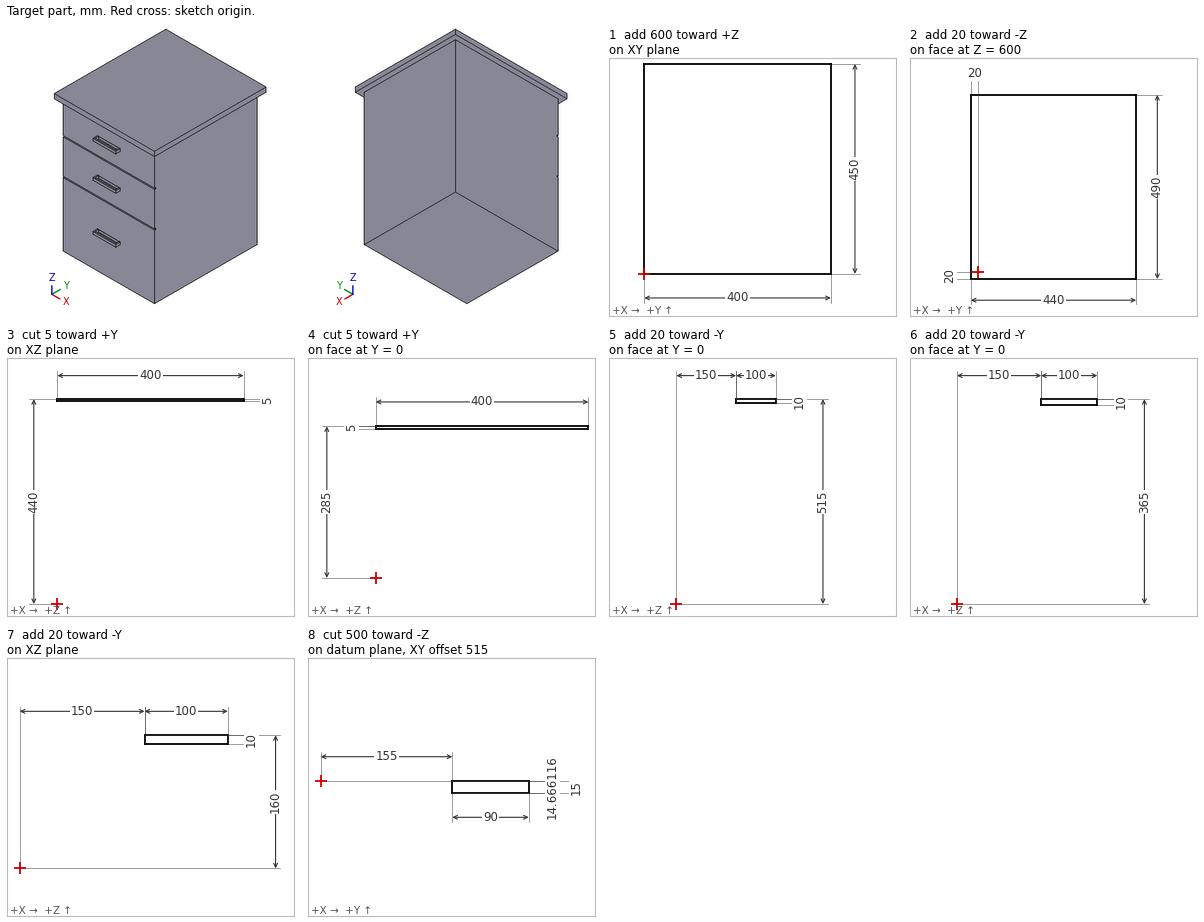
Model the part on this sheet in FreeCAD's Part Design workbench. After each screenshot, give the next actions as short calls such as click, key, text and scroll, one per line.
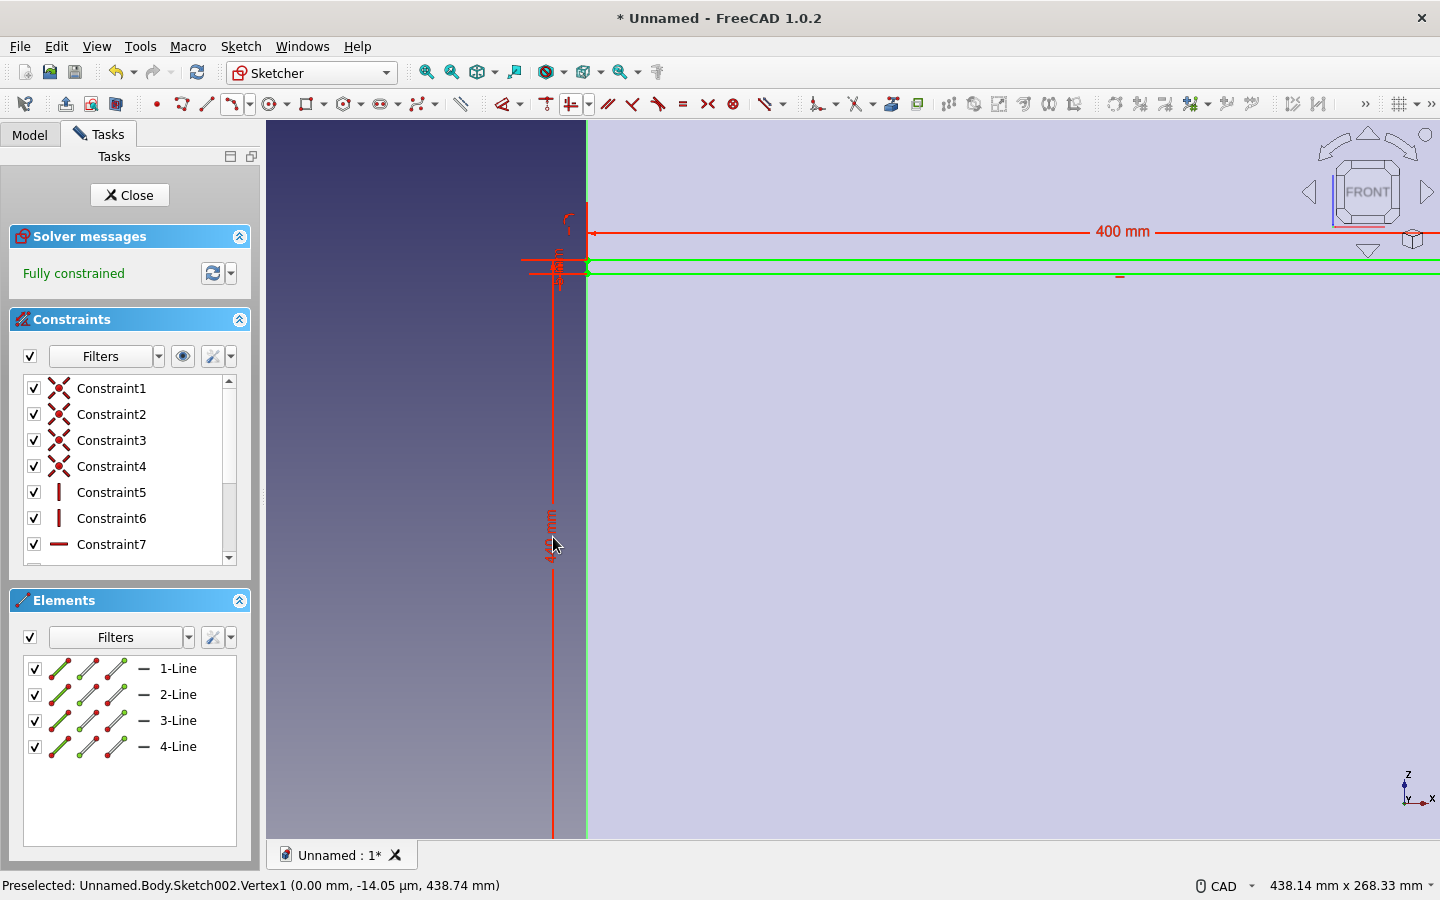
click(130, 195)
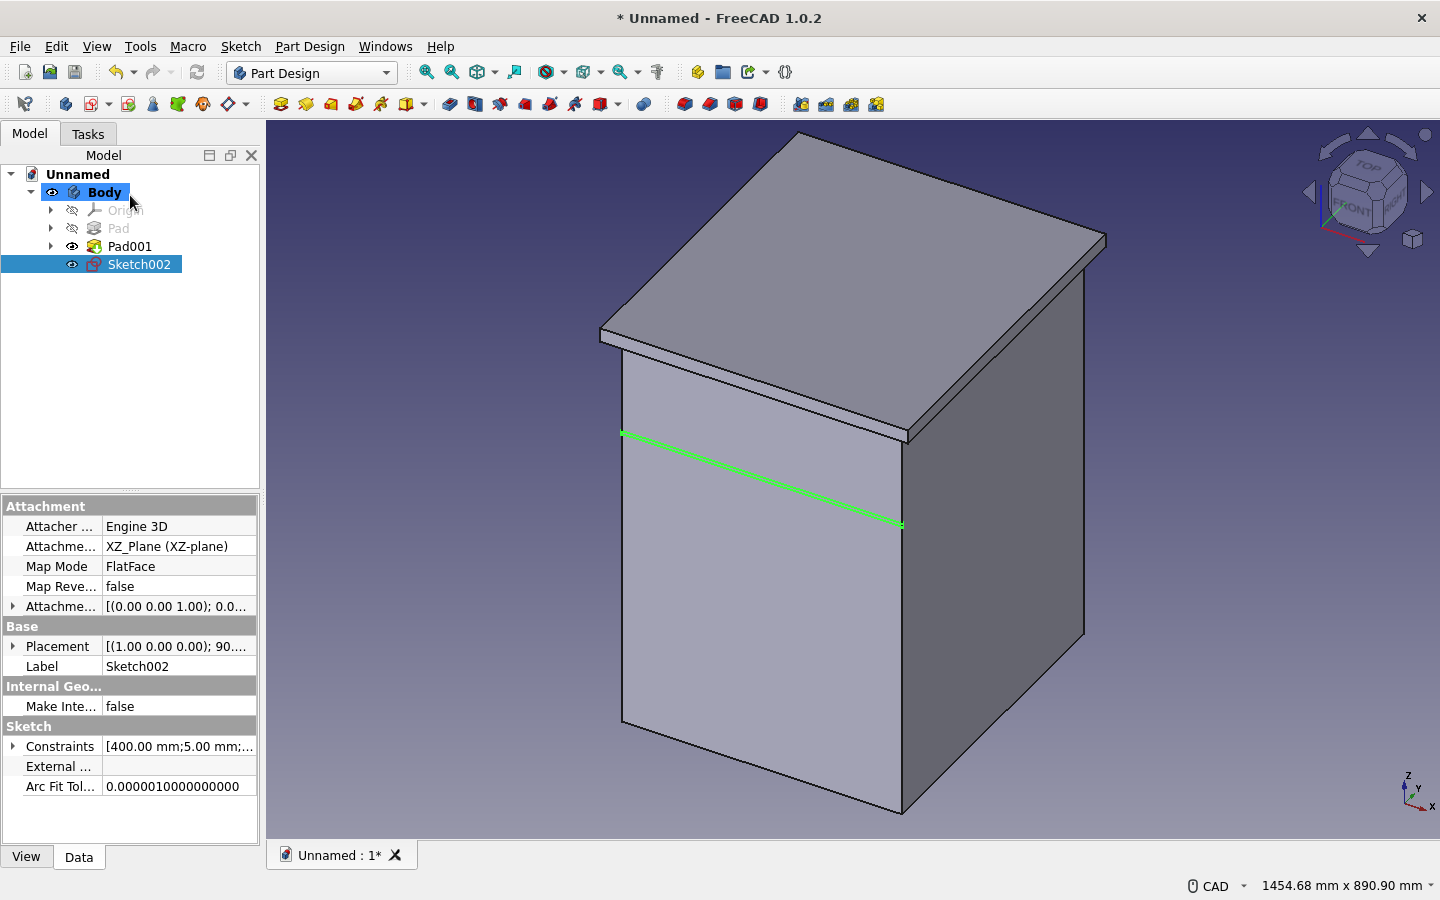
click(450, 104)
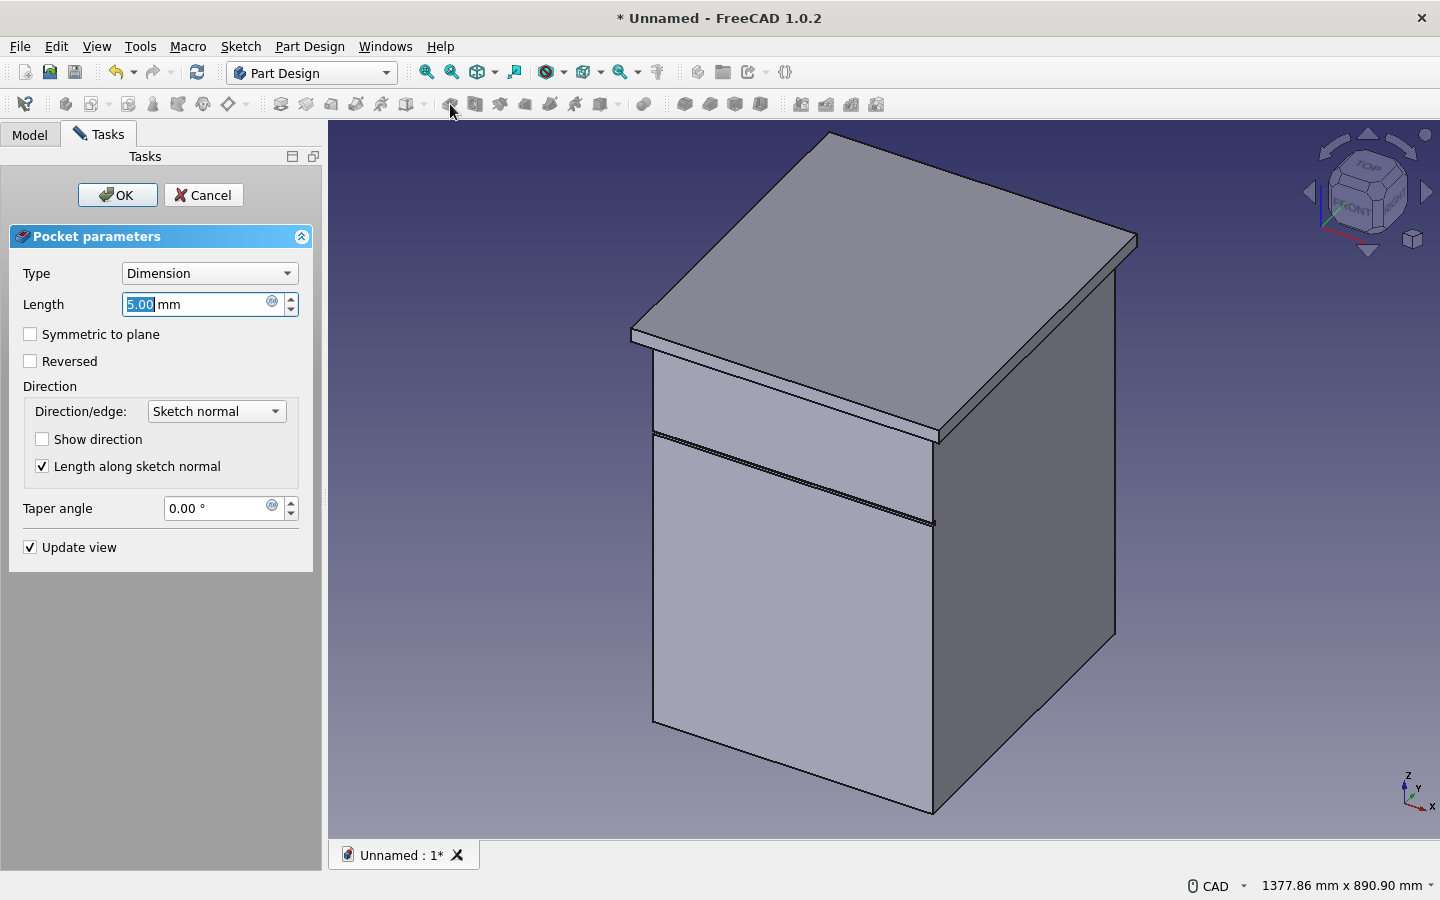
text(5)
key(Tab)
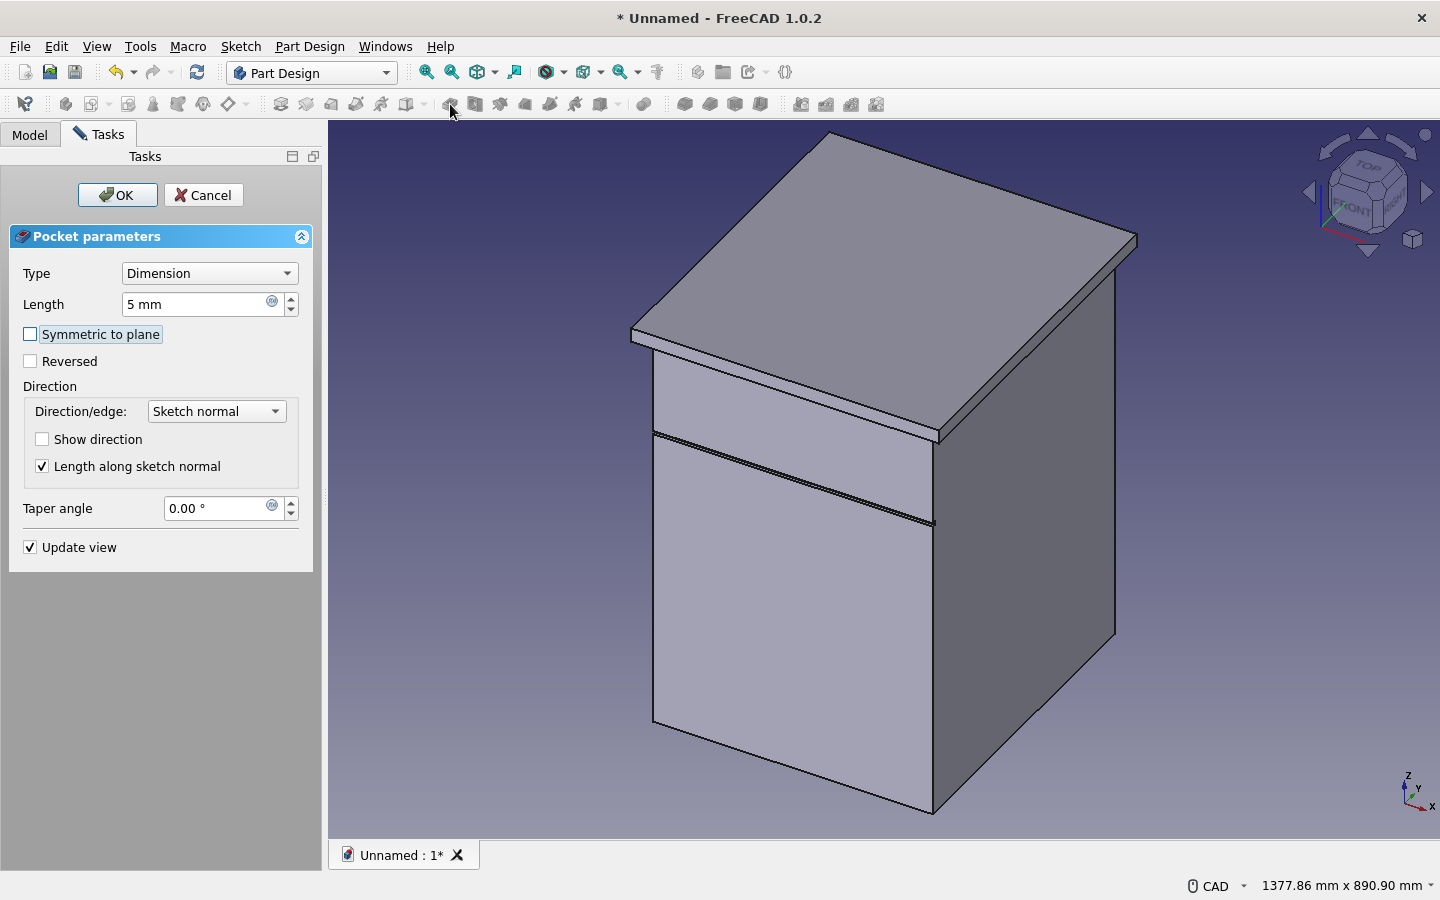
click(118, 195)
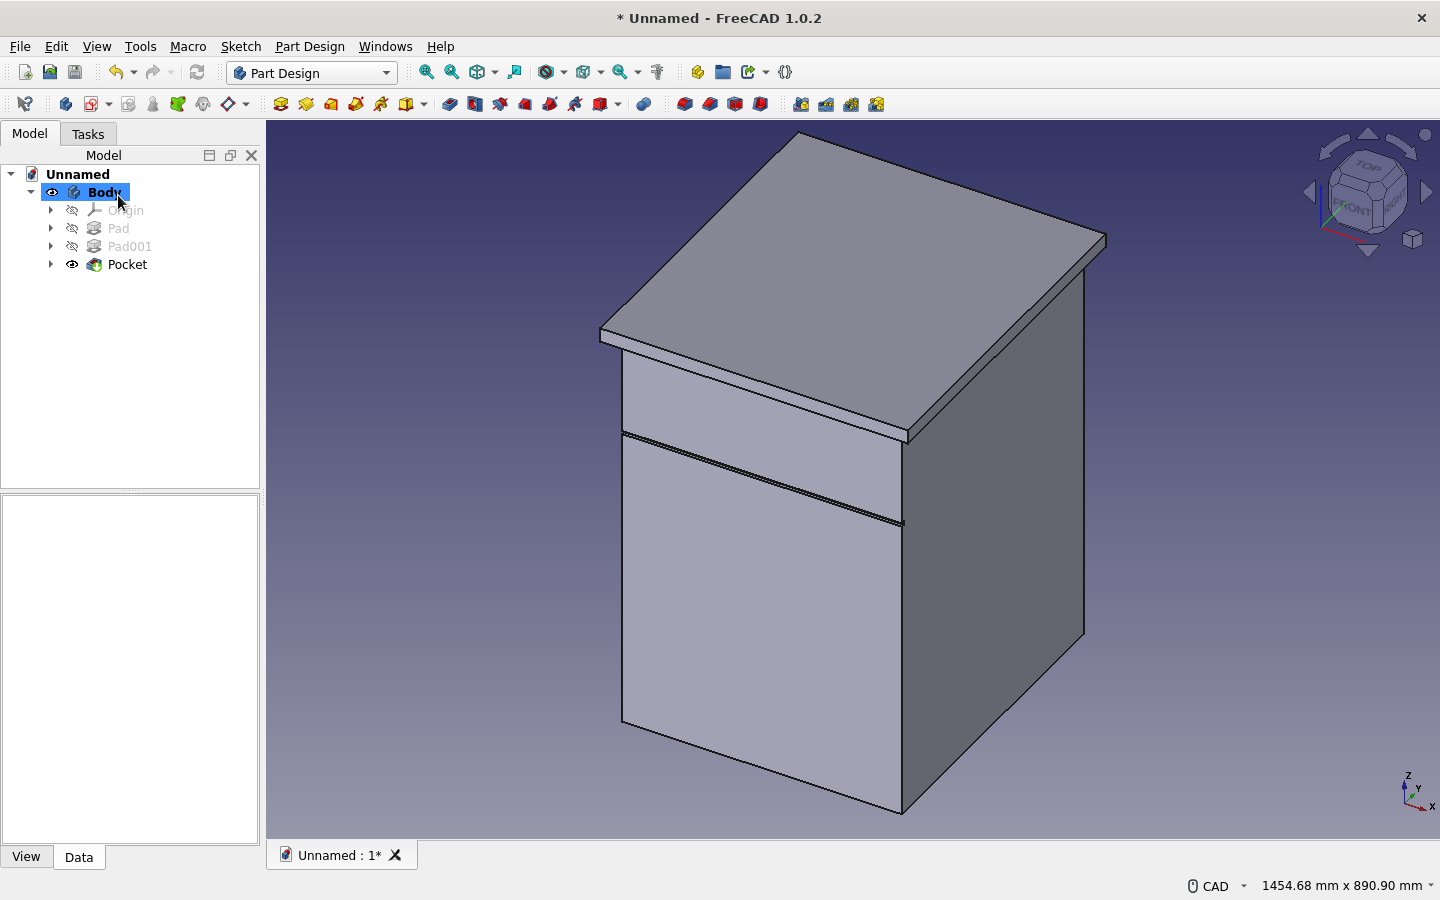
click(762, 623)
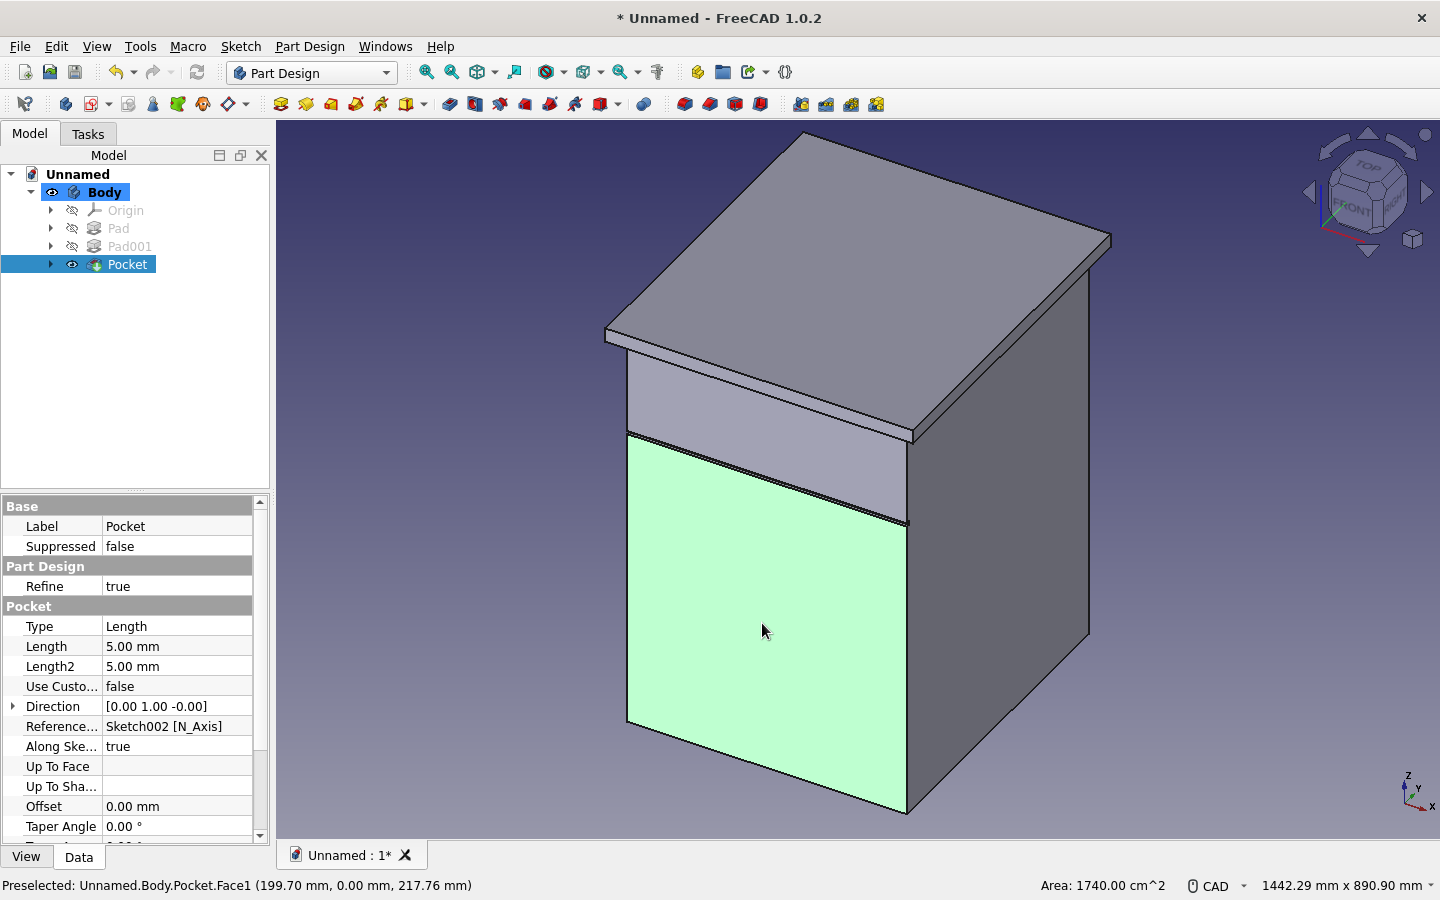
click(90, 104)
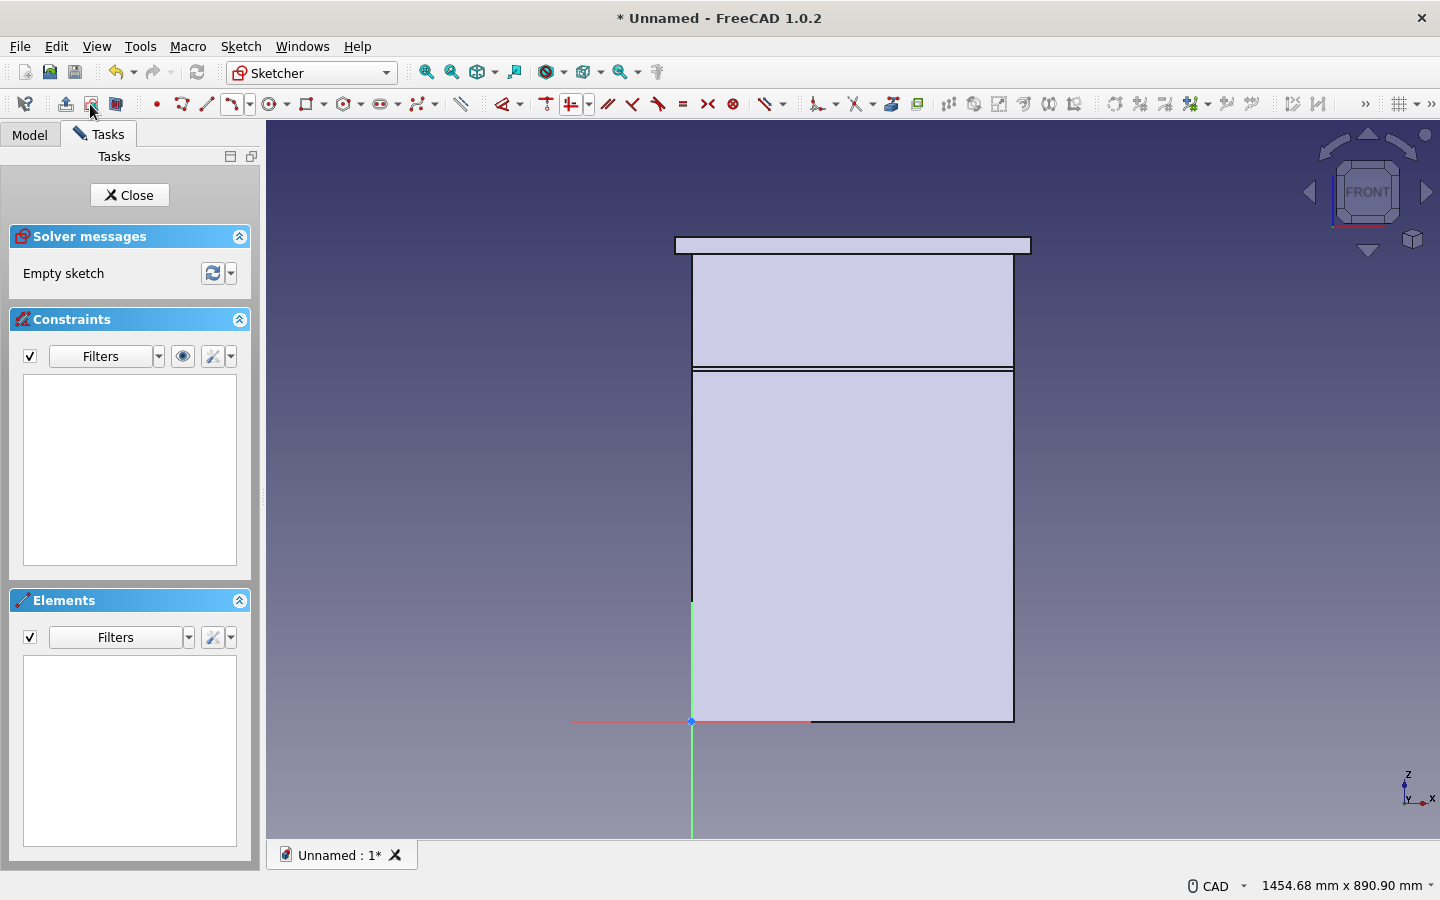
click(116, 104)